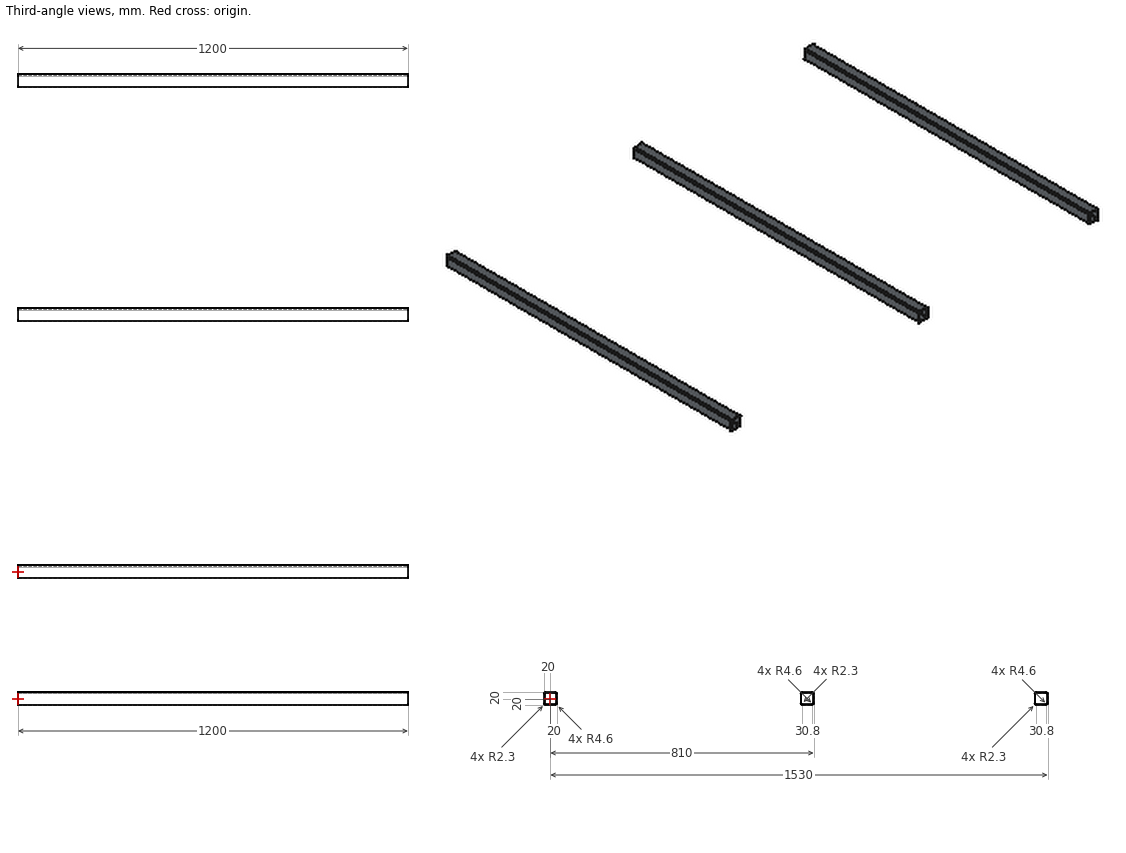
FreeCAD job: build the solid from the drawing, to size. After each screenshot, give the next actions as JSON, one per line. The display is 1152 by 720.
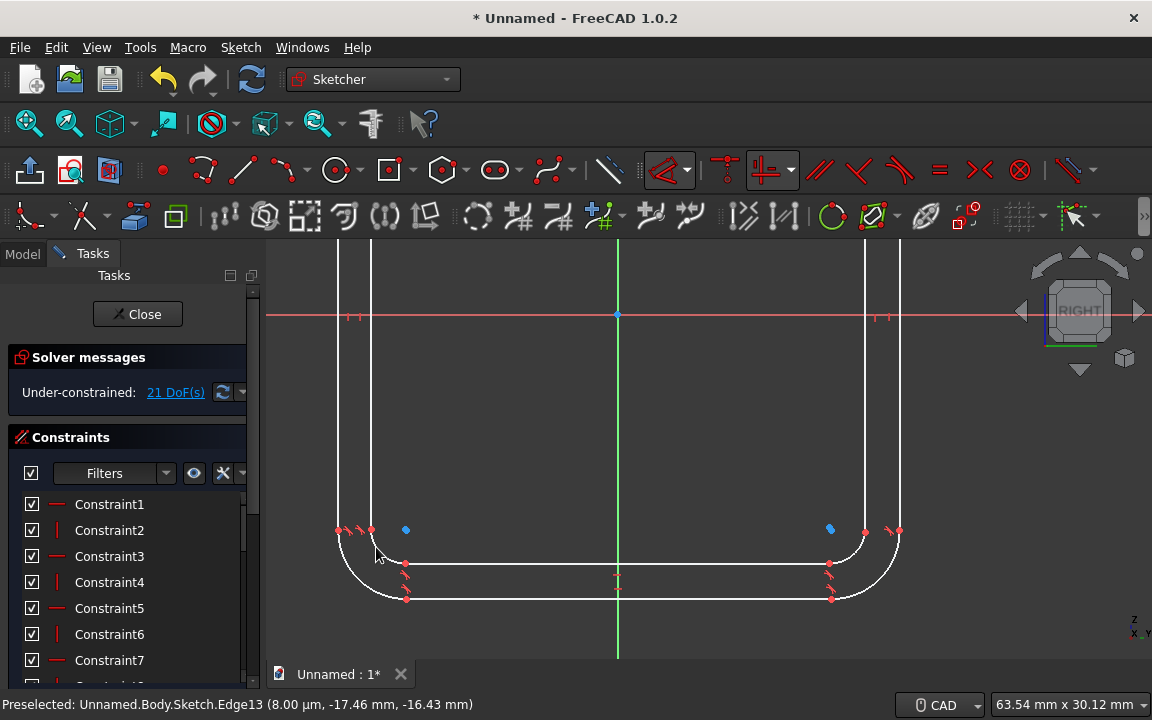
{"action": "left_click", "coordinate": [371, 401]}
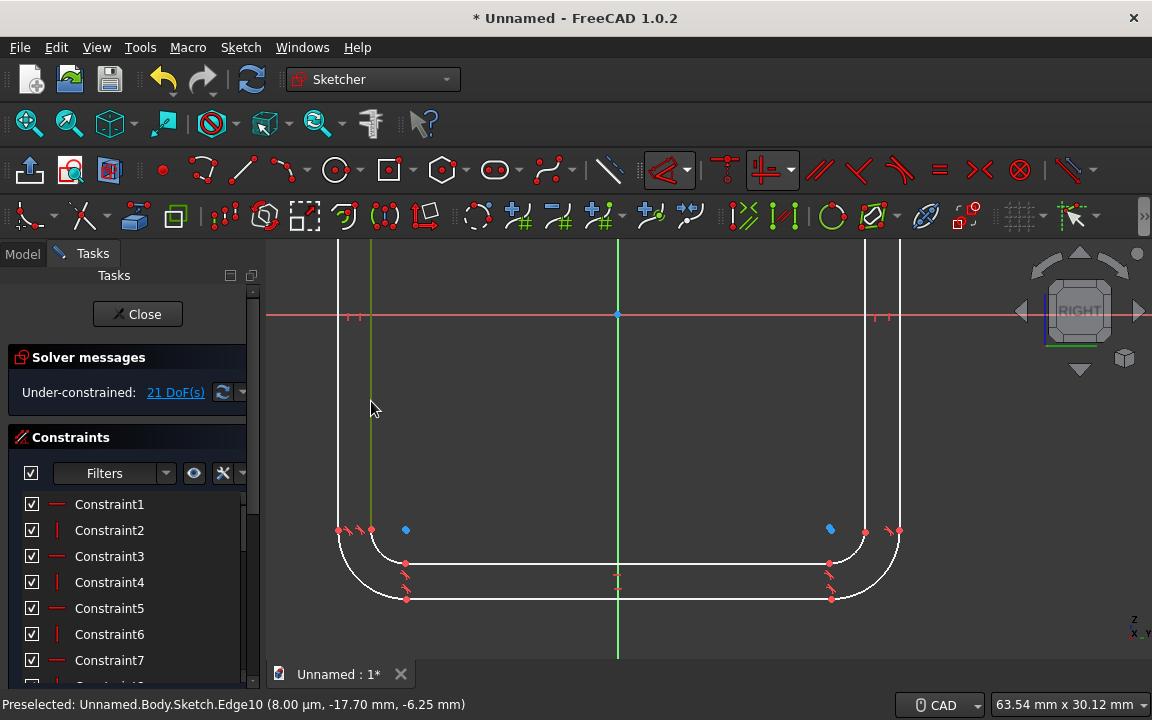
{"action": "scroll", "coordinate": [659, 558], "scroll_direction": "down", "scroll_amount": 4}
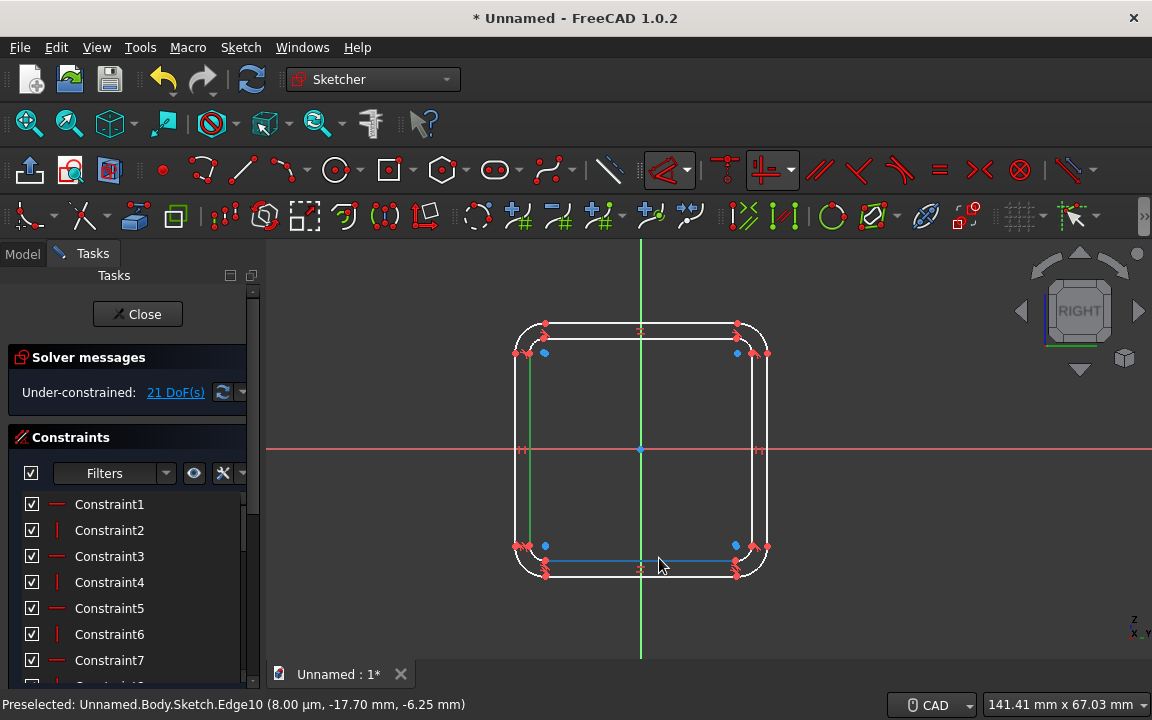
{"action": "scroll", "coordinate": [537, 341], "scroll_direction": "up", "scroll_amount": 4}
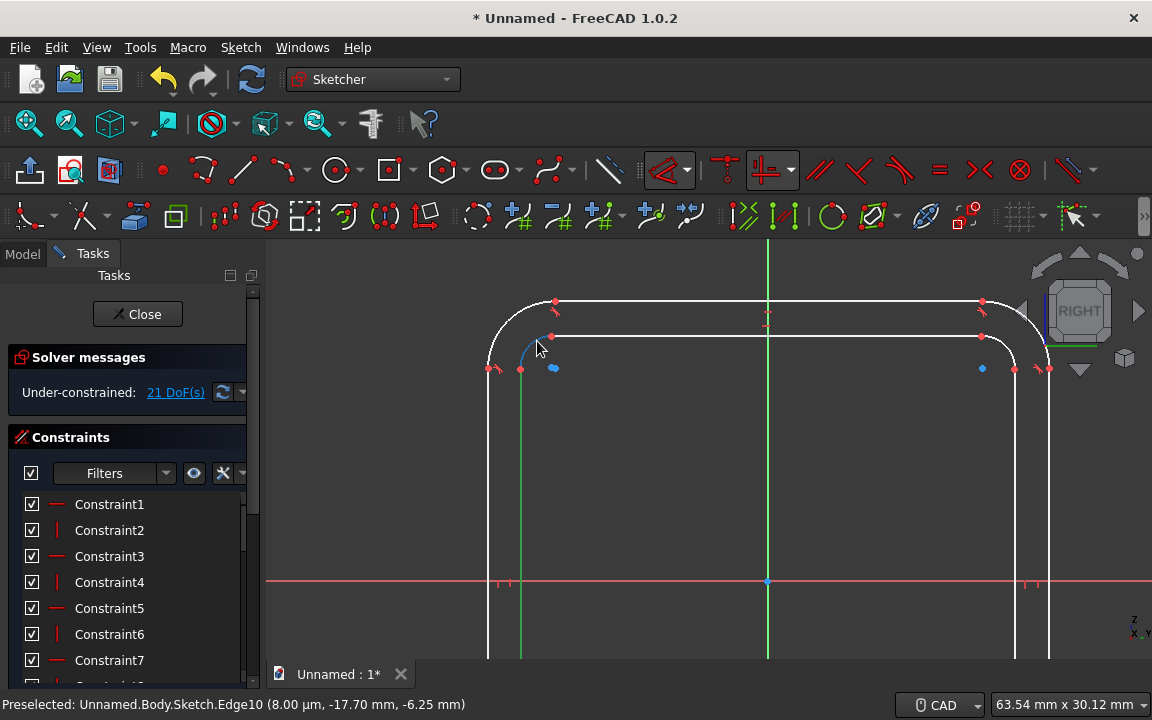
{"action": "left_click", "coordinate": [537, 340]}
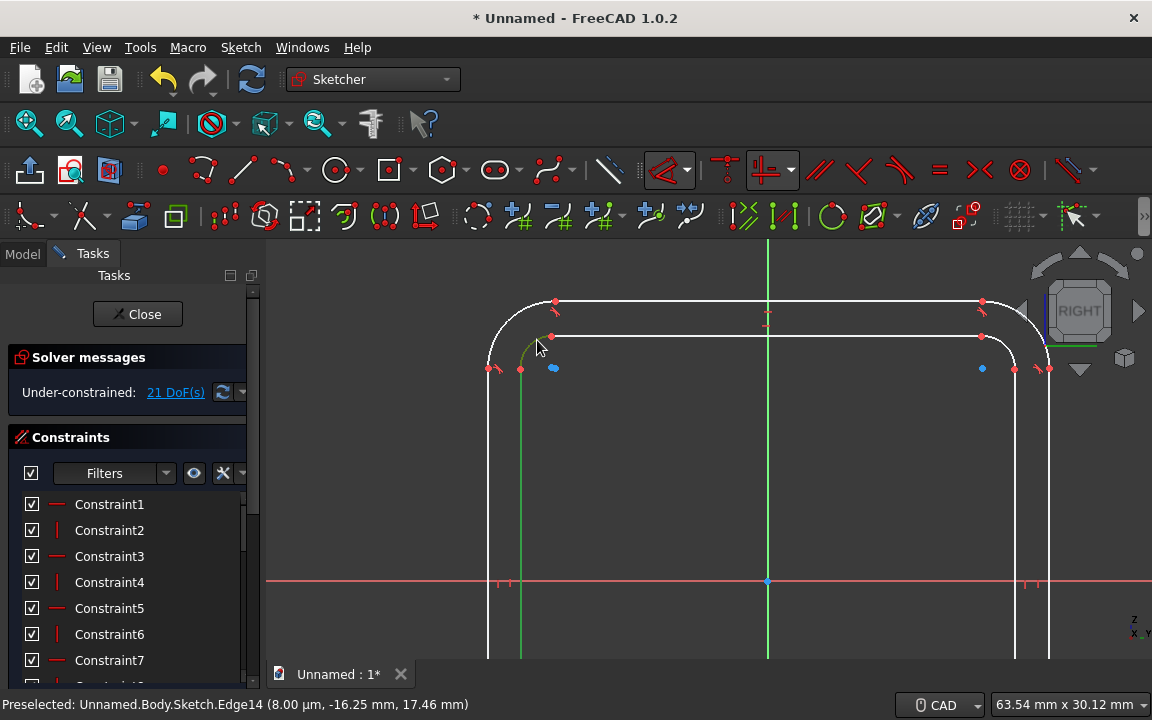
{"action": "key", "text": "t"}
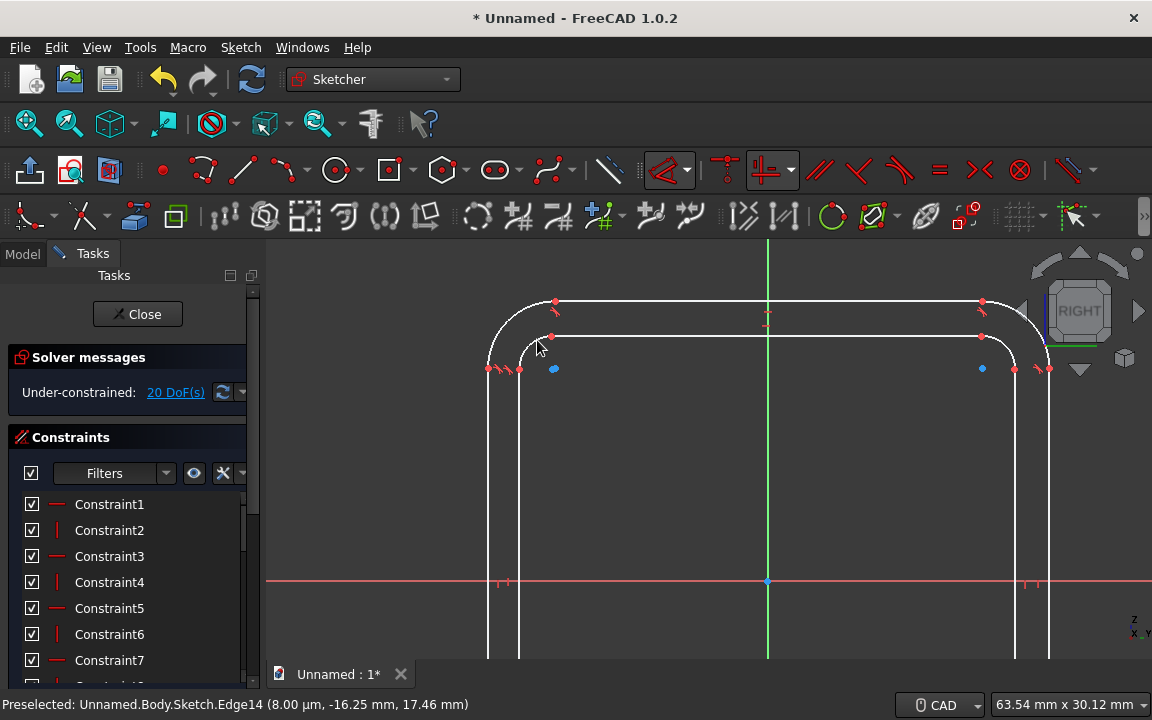
{"action": "left_click", "coordinate": [681, 336]}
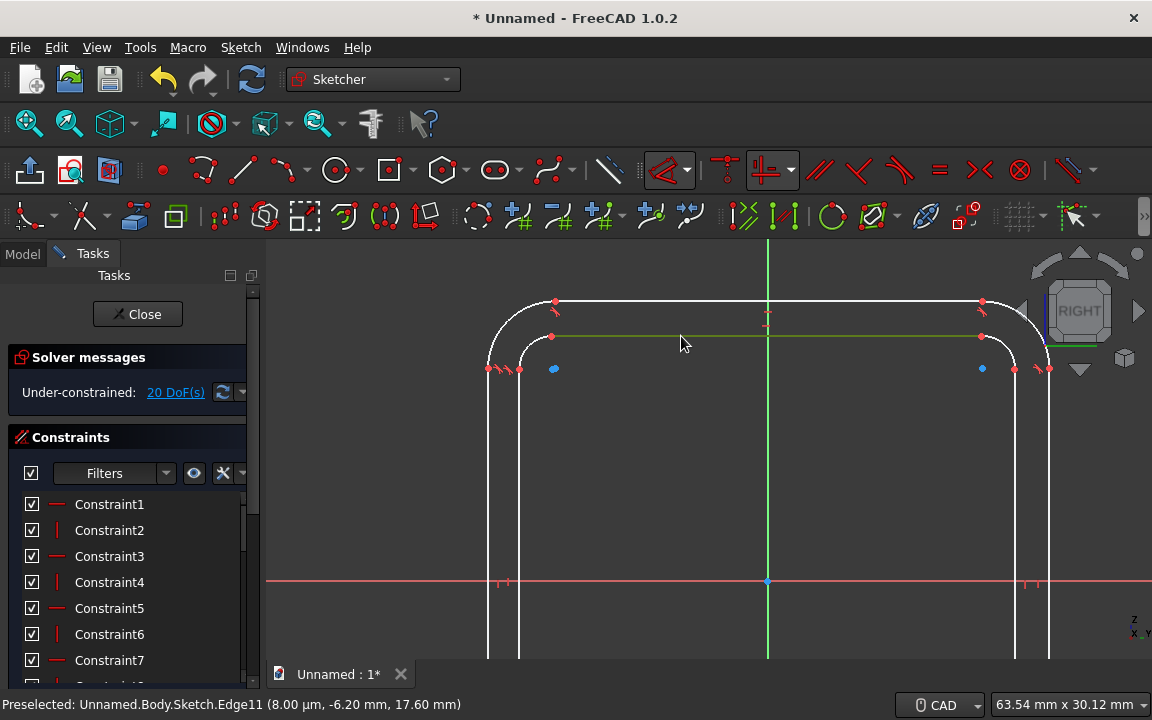
{"action": "left_click", "coordinate": [537, 340]}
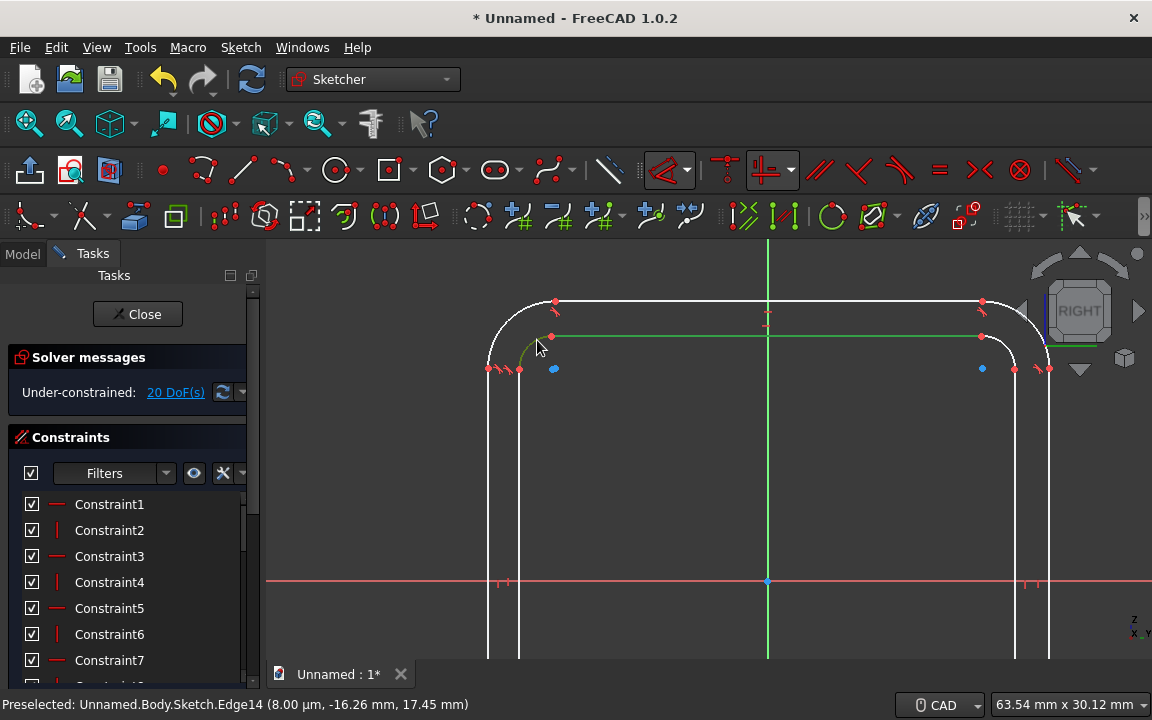
{"action": "left_click", "coordinate": [900, 170]}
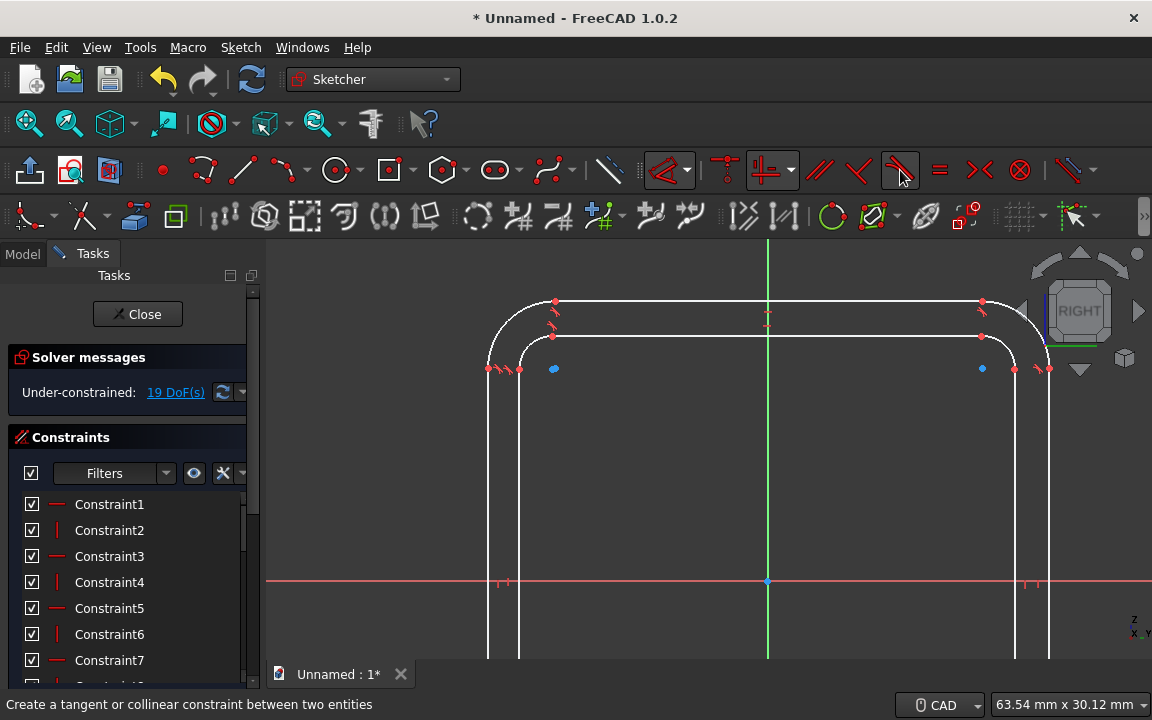
{"action": "left_click", "coordinate": [681, 336]}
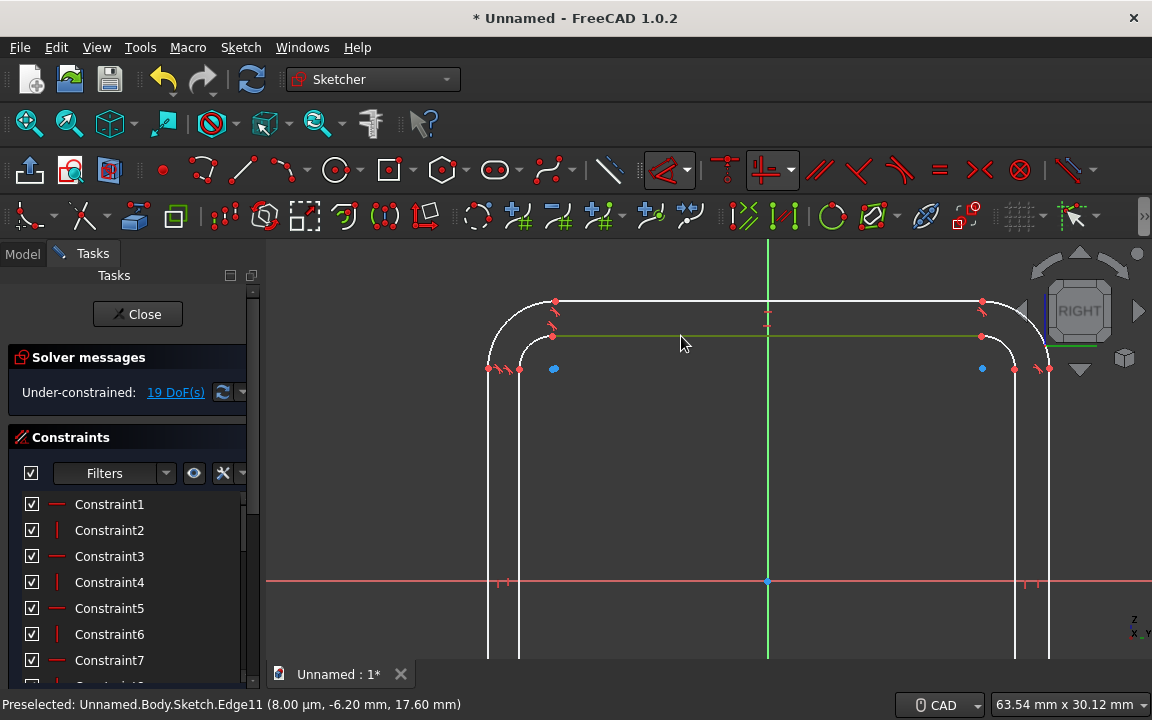
{"action": "scroll", "coordinate": [537, 341], "scroll_direction": "down", "scroll_amount": 4}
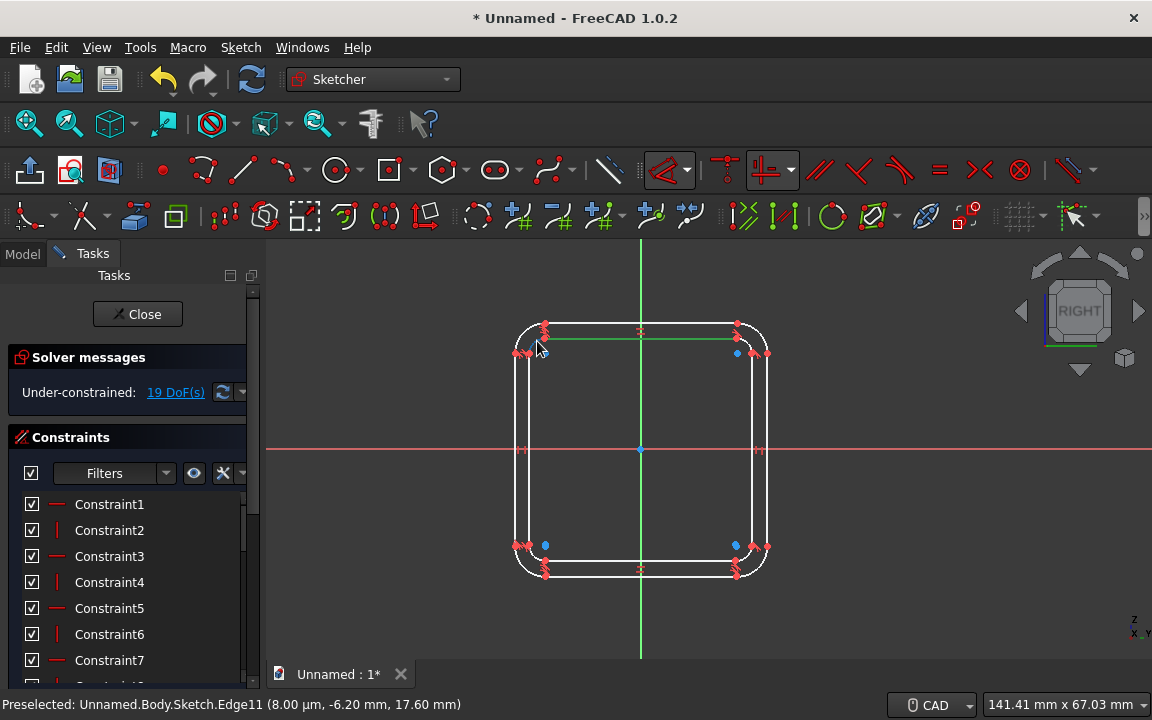
{"action": "scroll", "coordinate": [750, 347], "scroll_direction": "up", "scroll_amount": 4}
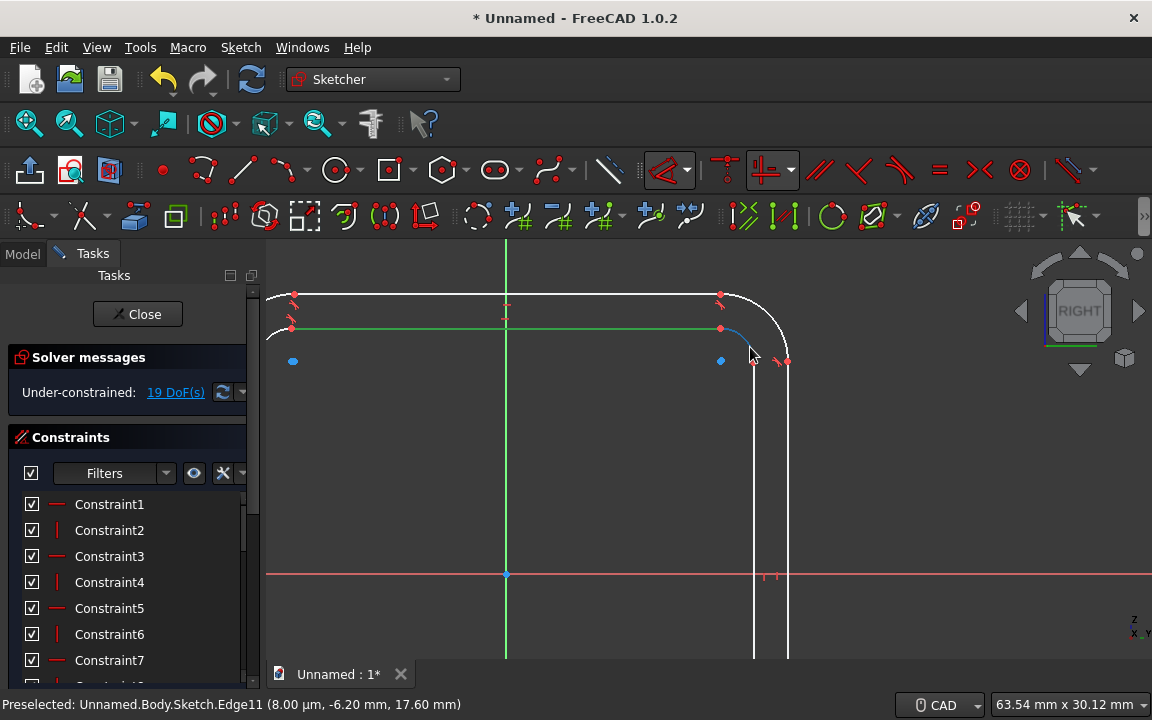
{"action": "left_click", "coordinate": [750, 347]}